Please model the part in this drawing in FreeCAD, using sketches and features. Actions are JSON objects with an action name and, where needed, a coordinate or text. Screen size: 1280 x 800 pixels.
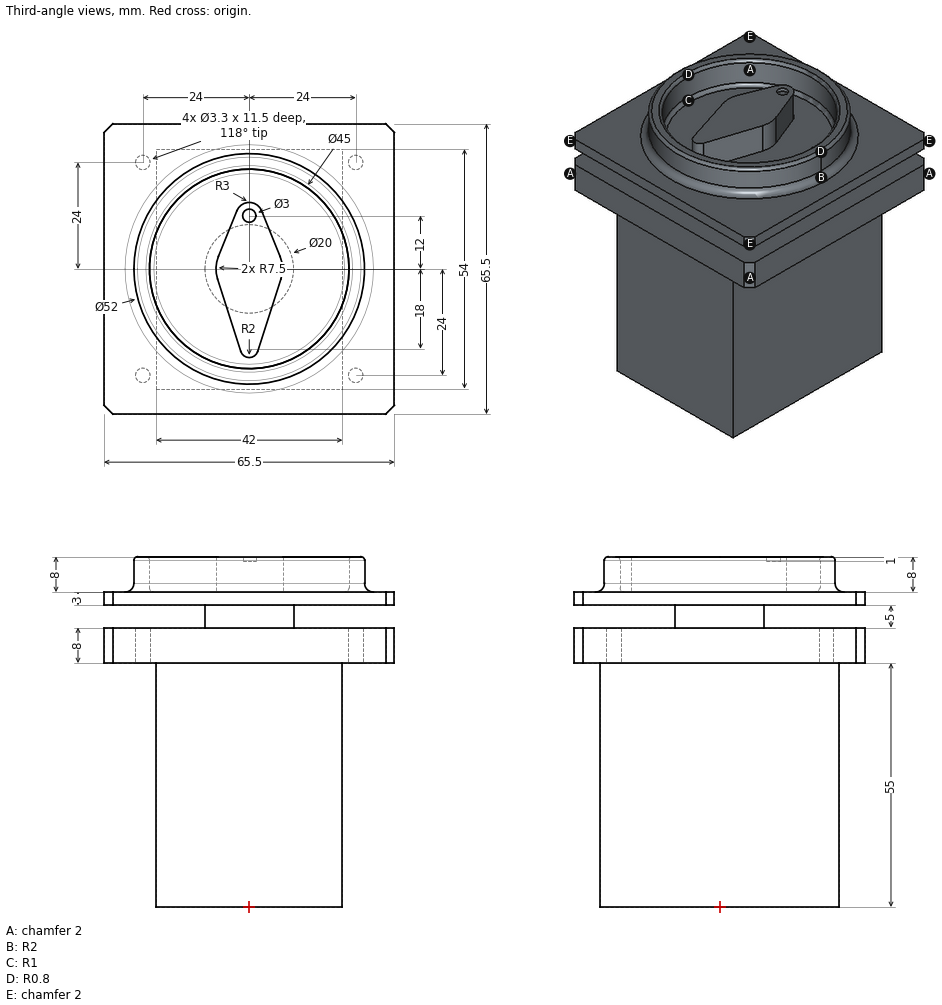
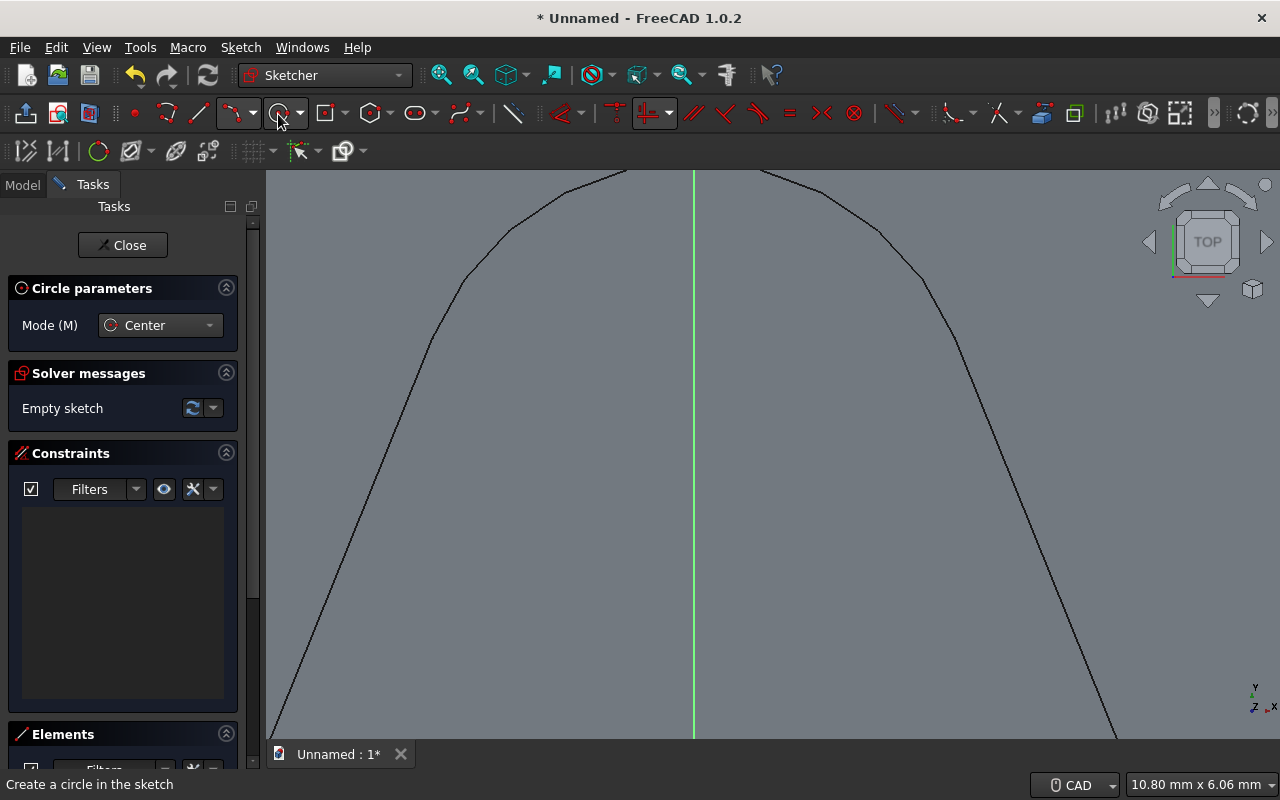
{"action": "left_click", "coordinate": [694, 444]}
{"action": "mouse_move", "coordinate": [793, 344]}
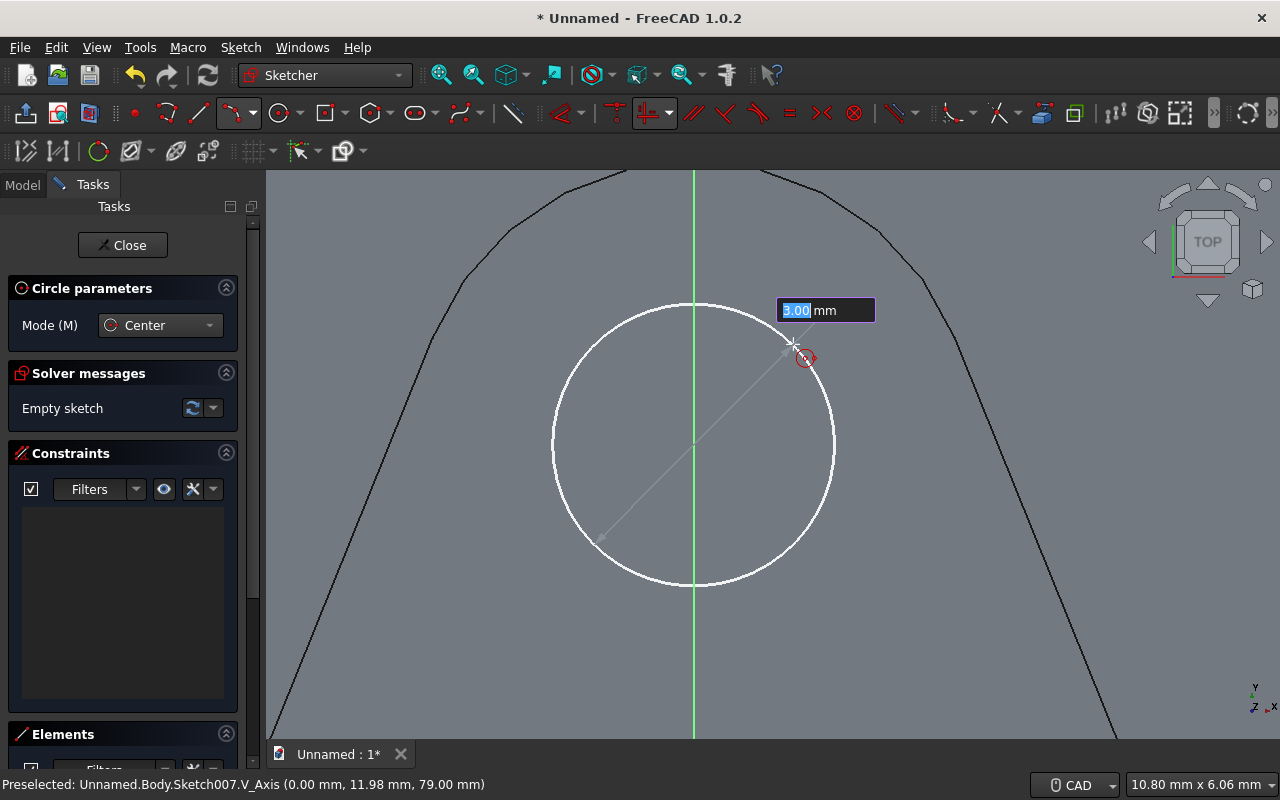
{"action": "type", "text": "3"}
{"action": "key", "text": "Return"}
{"action": "key", "text": "Escape"}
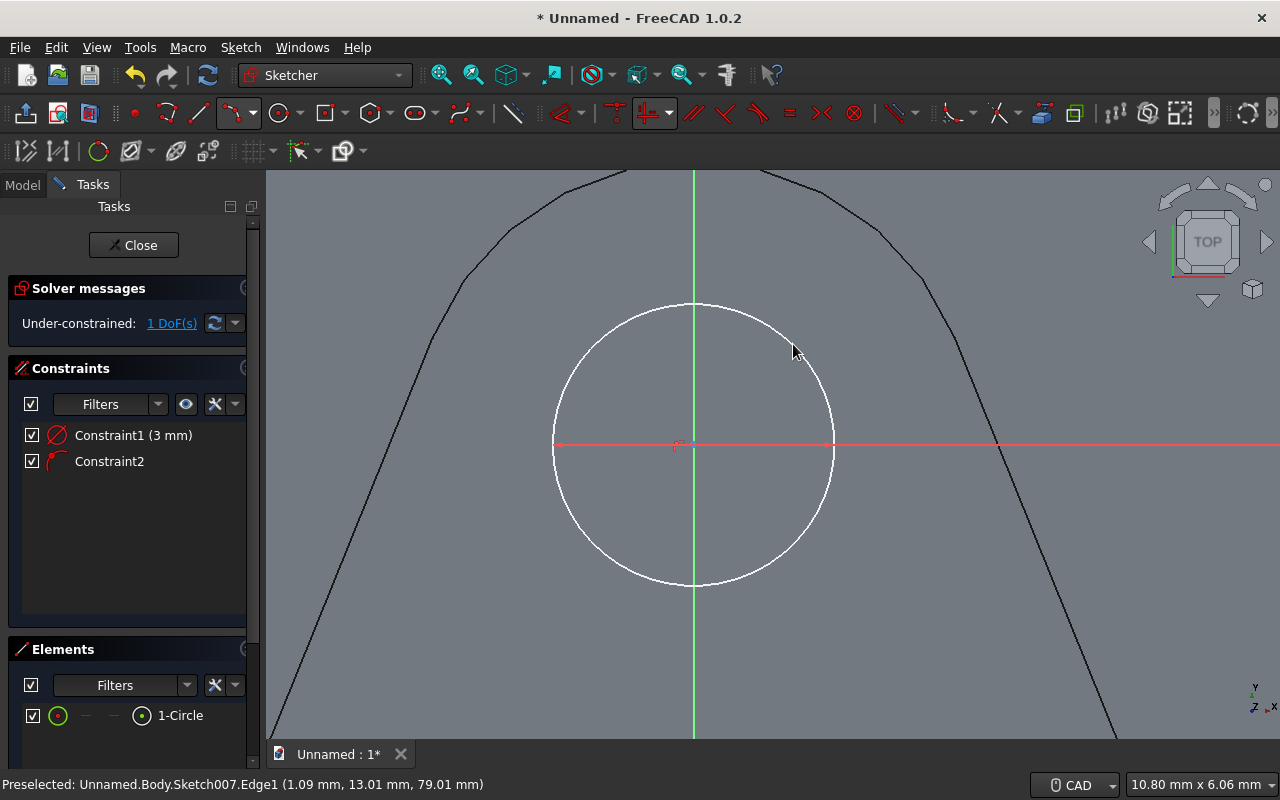
{"action": "left_click", "coordinate": [560, 114]}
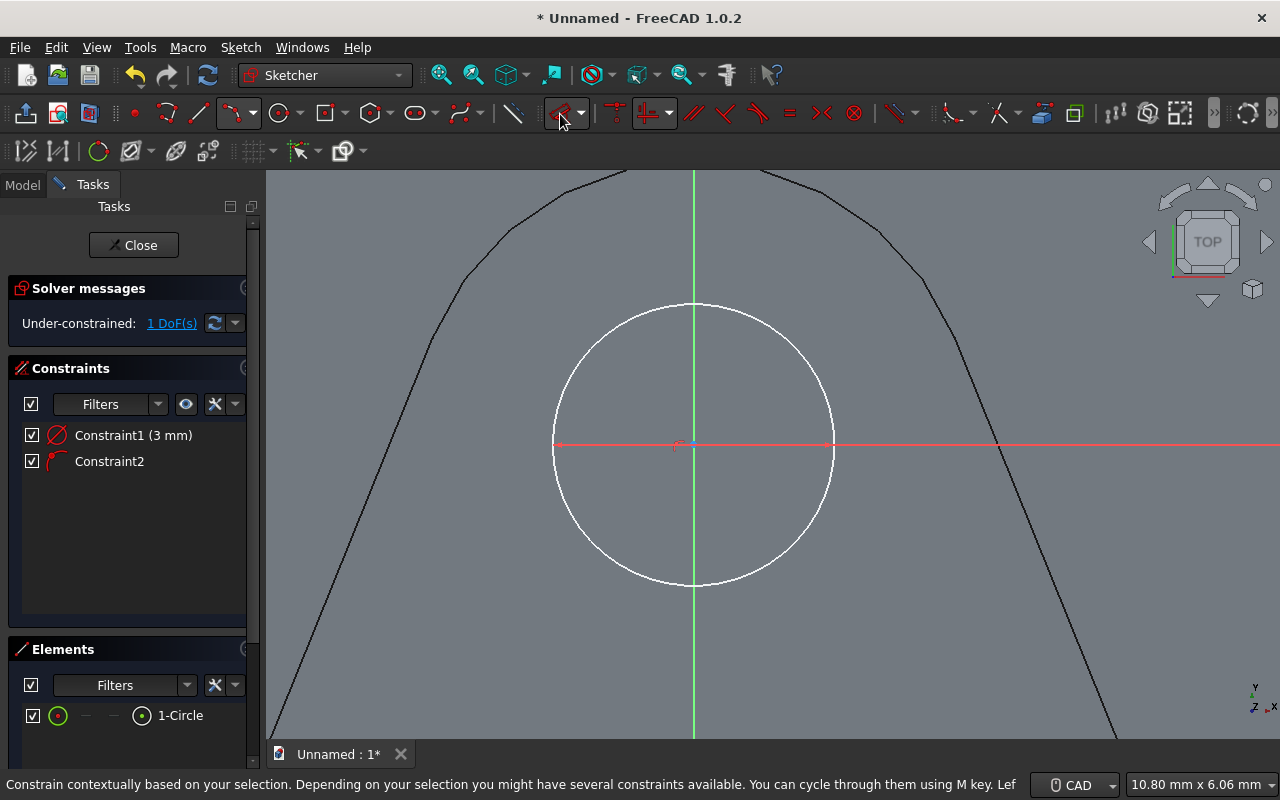
{"action": "left_click", "coordinate": [694, 445]}
{"action": "left_click", "coordinate": [728, 517]}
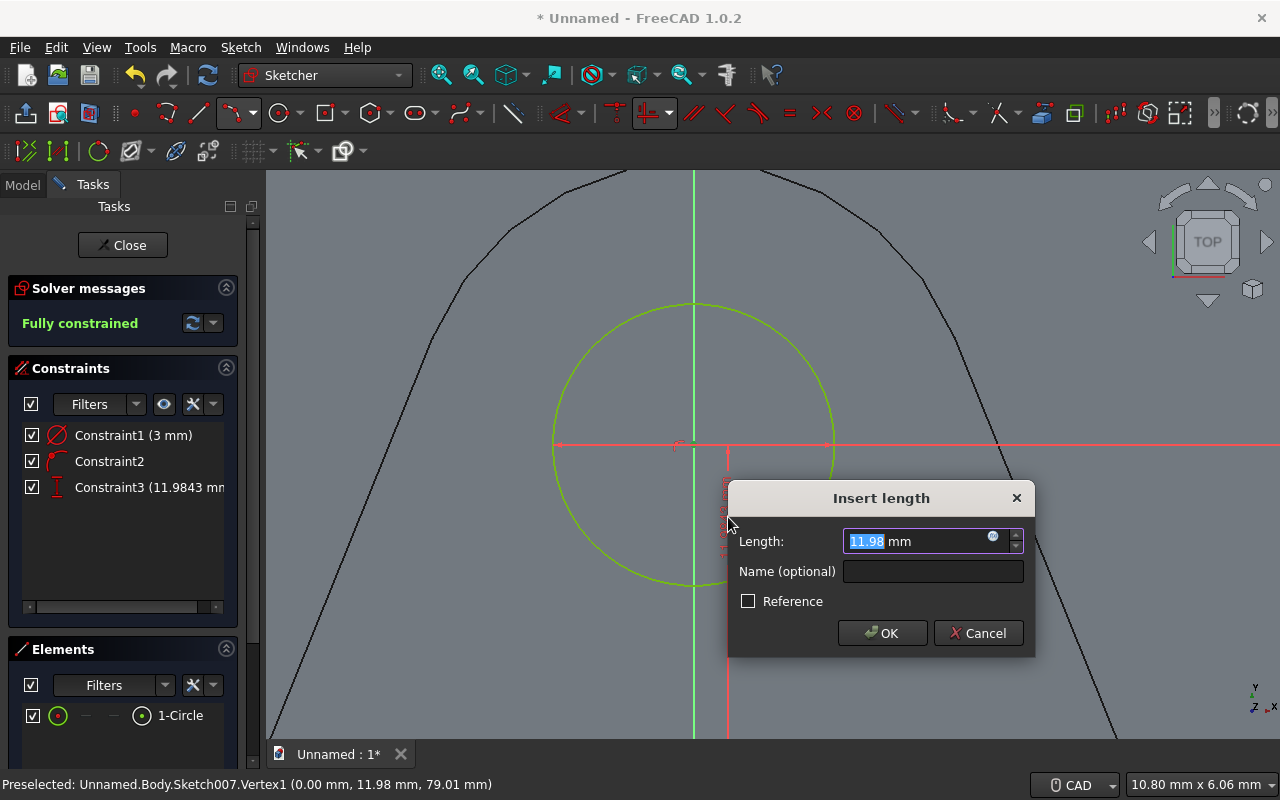
{"action": "type", "text": "12"}
{"action": "key", "text": "Return"}
{"action": "key", "text": "Escape"}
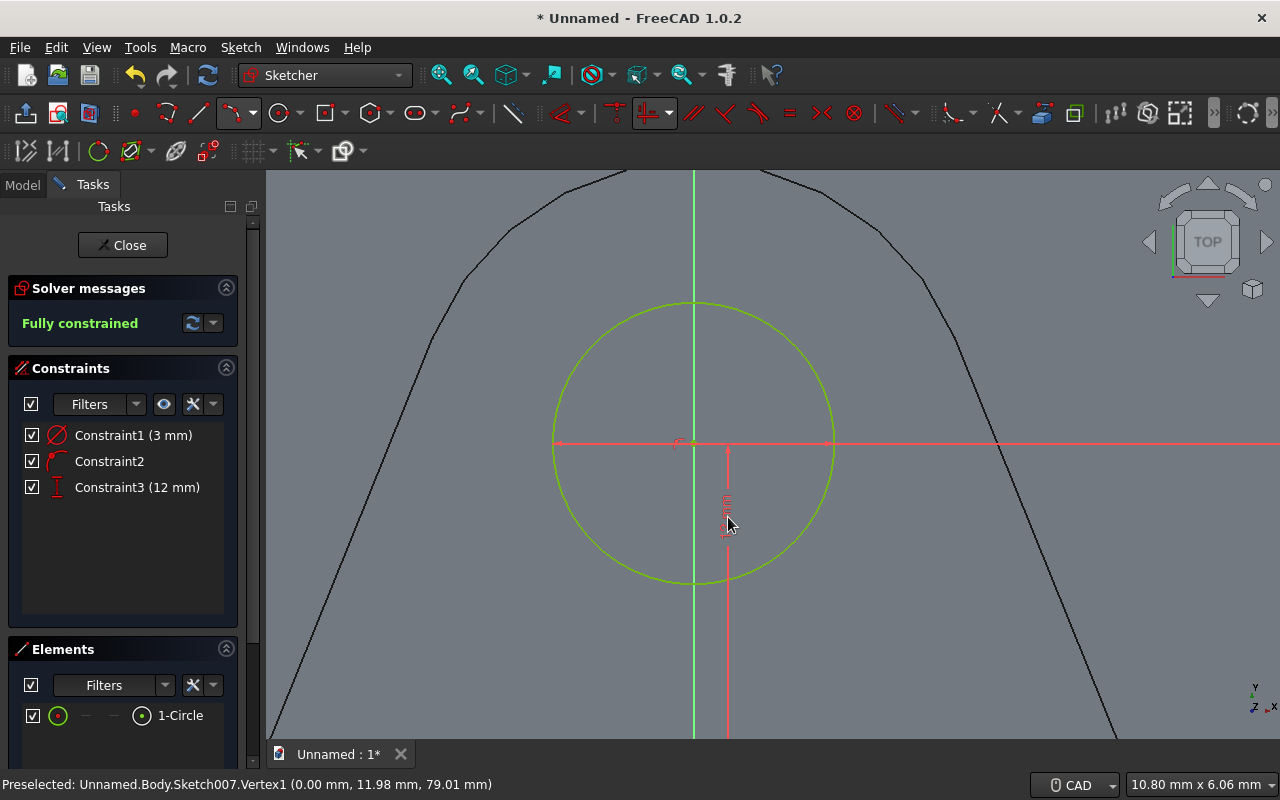
{"action": "left_click", "coordinate": [123, 245]}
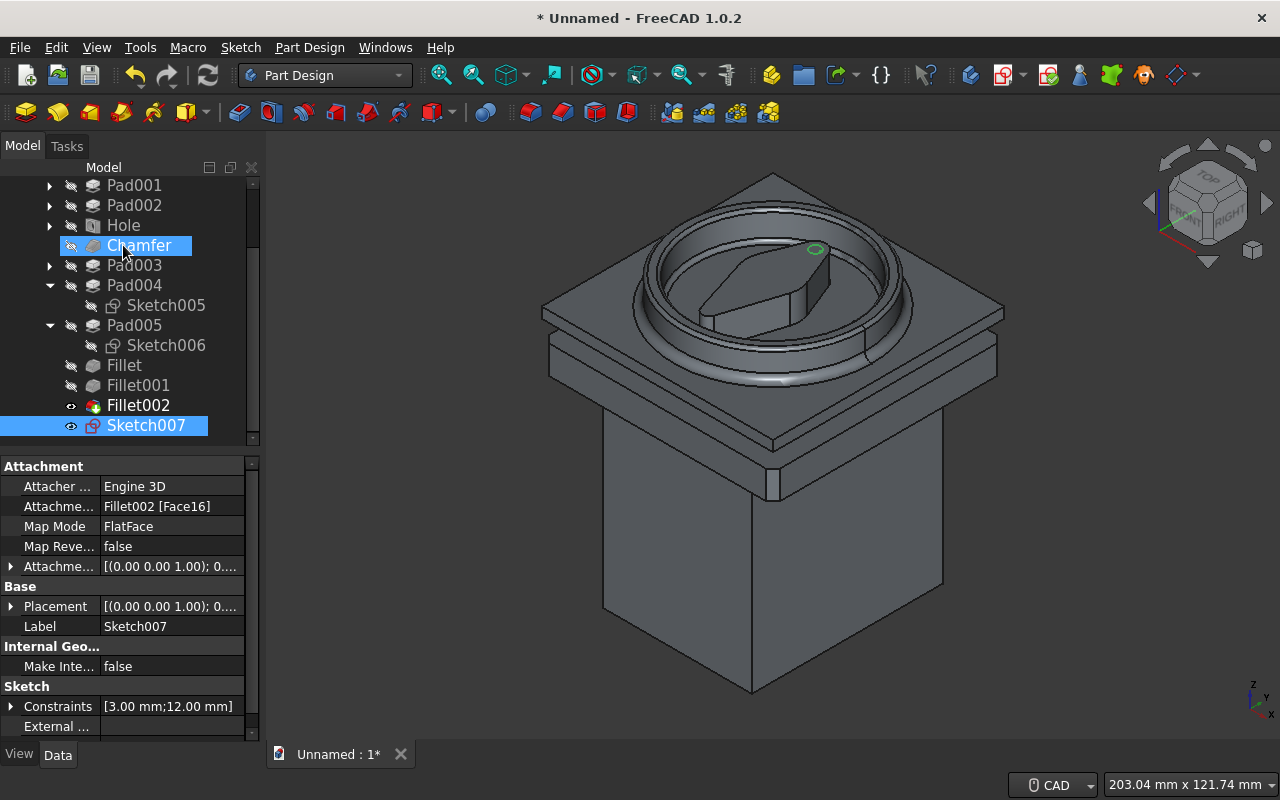
{"action": "left_click", "coordinate": [240, 112]}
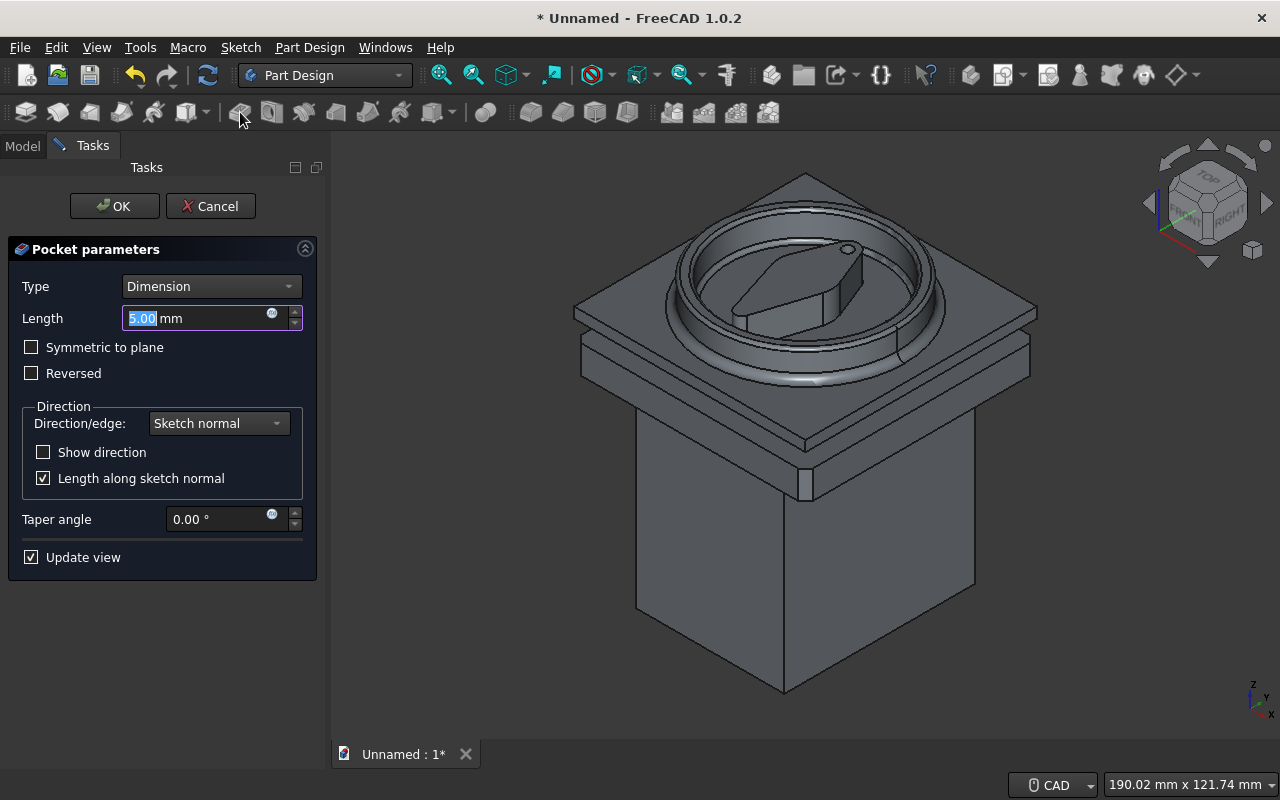
{"action": "type", "text": "1"}
{"action": "key", "text": "Tab"}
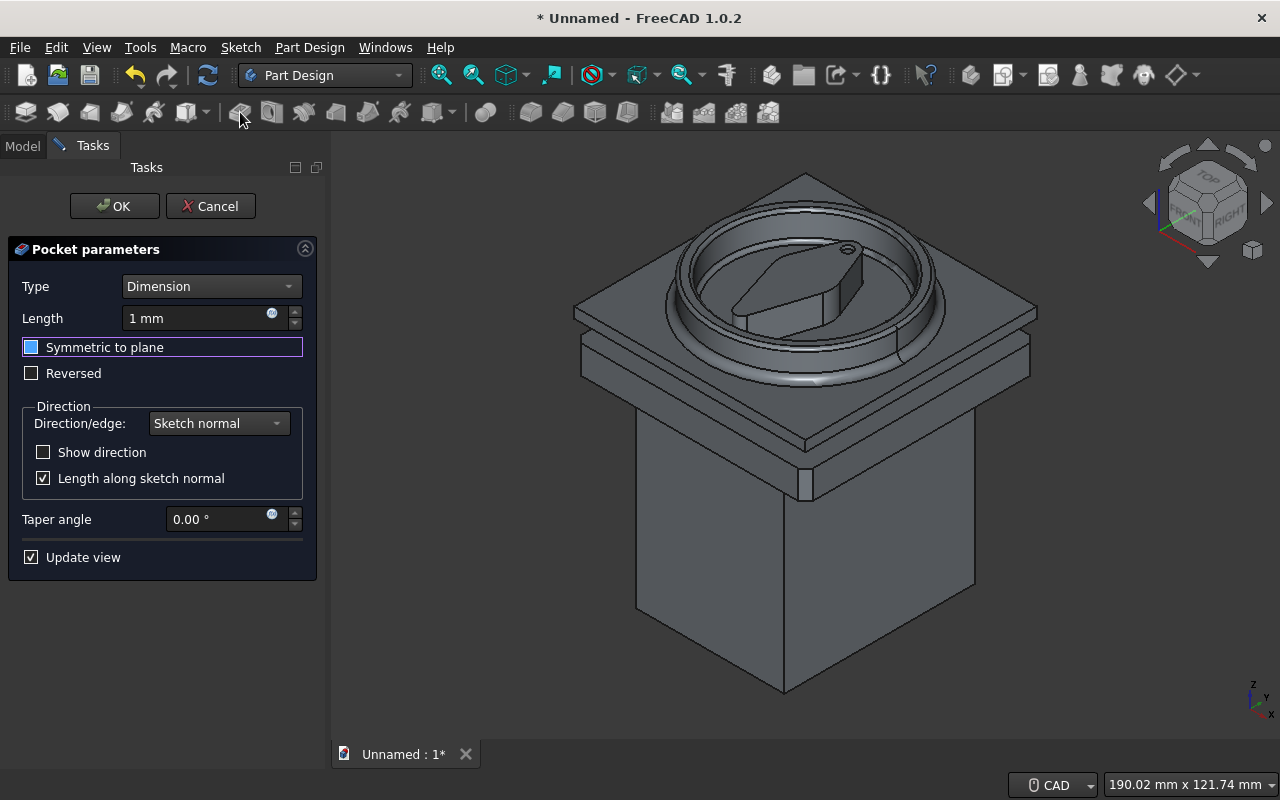
{"action": "left_click", "coordinate": [115, 206]}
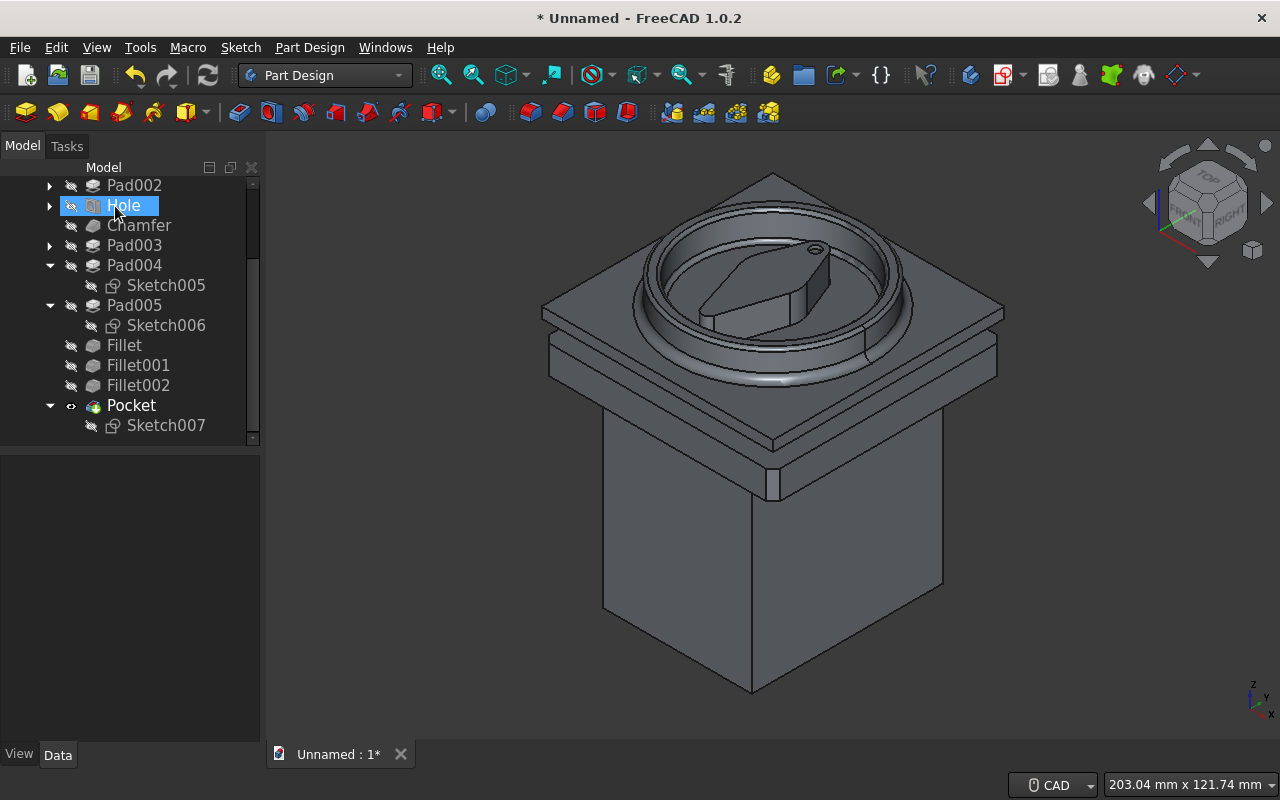
{"action": "left_click", "coordinate": [773, 445]}